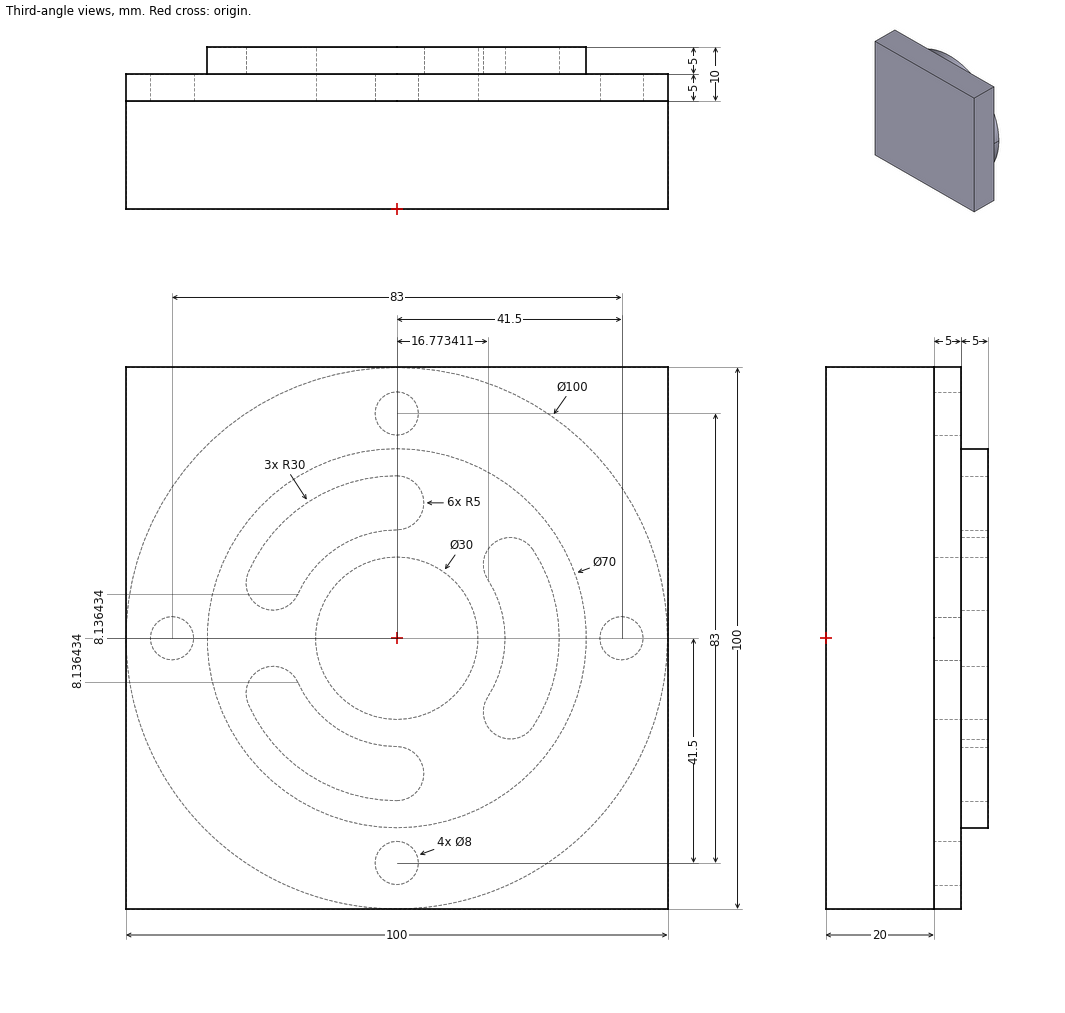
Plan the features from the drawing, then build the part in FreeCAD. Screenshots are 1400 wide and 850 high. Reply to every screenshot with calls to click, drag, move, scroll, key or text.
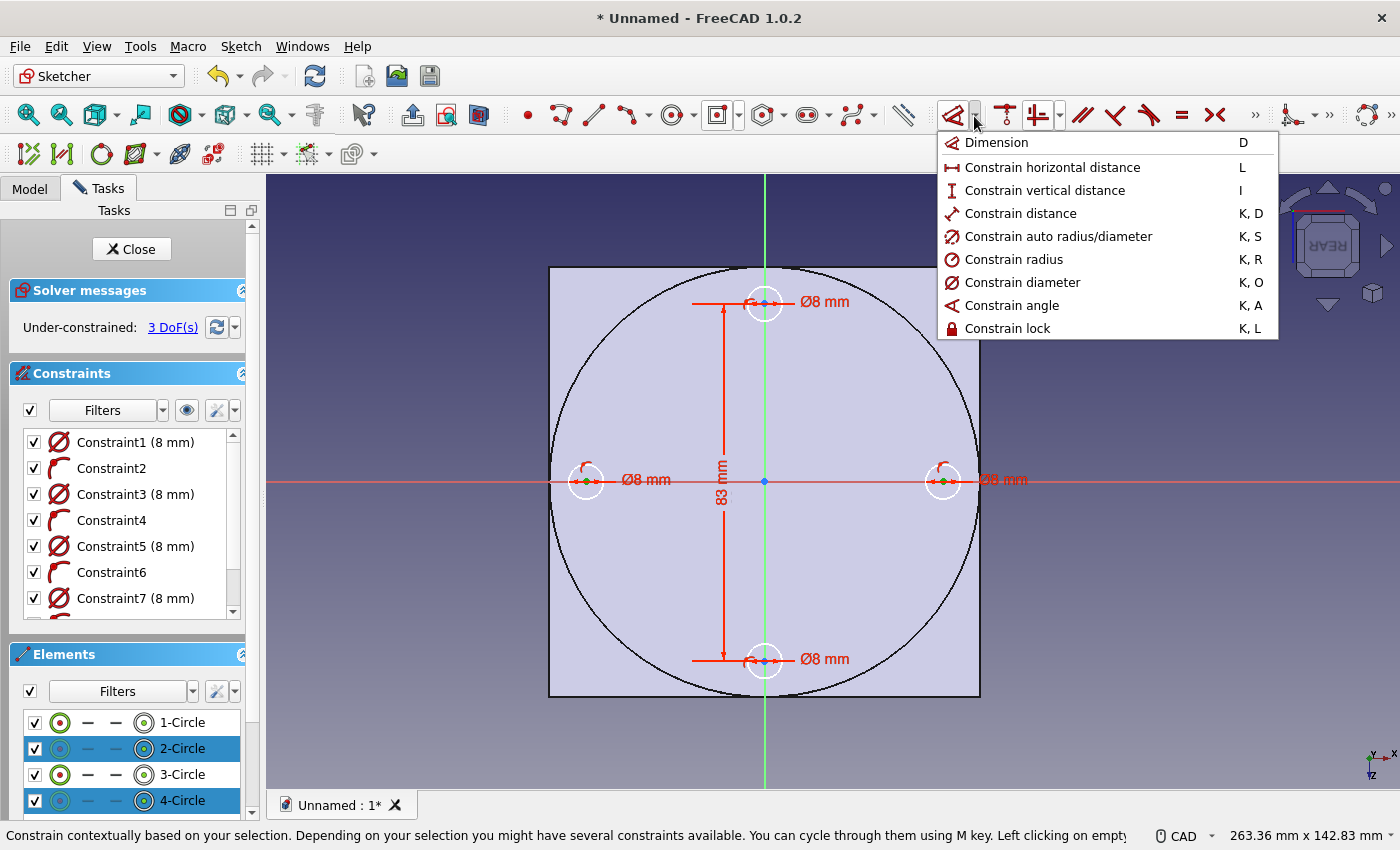
click(1108, 168)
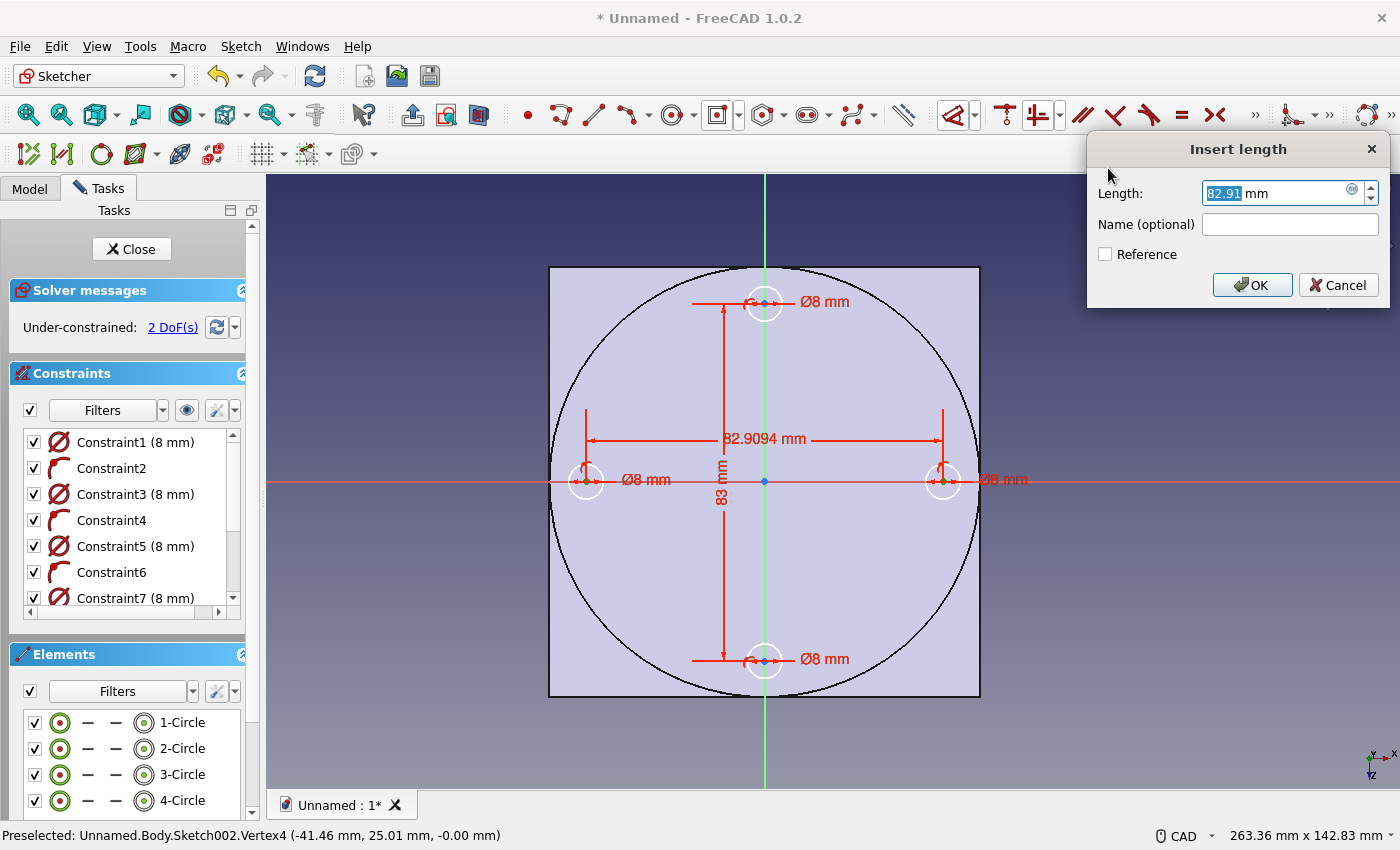
text(83)
key(Return)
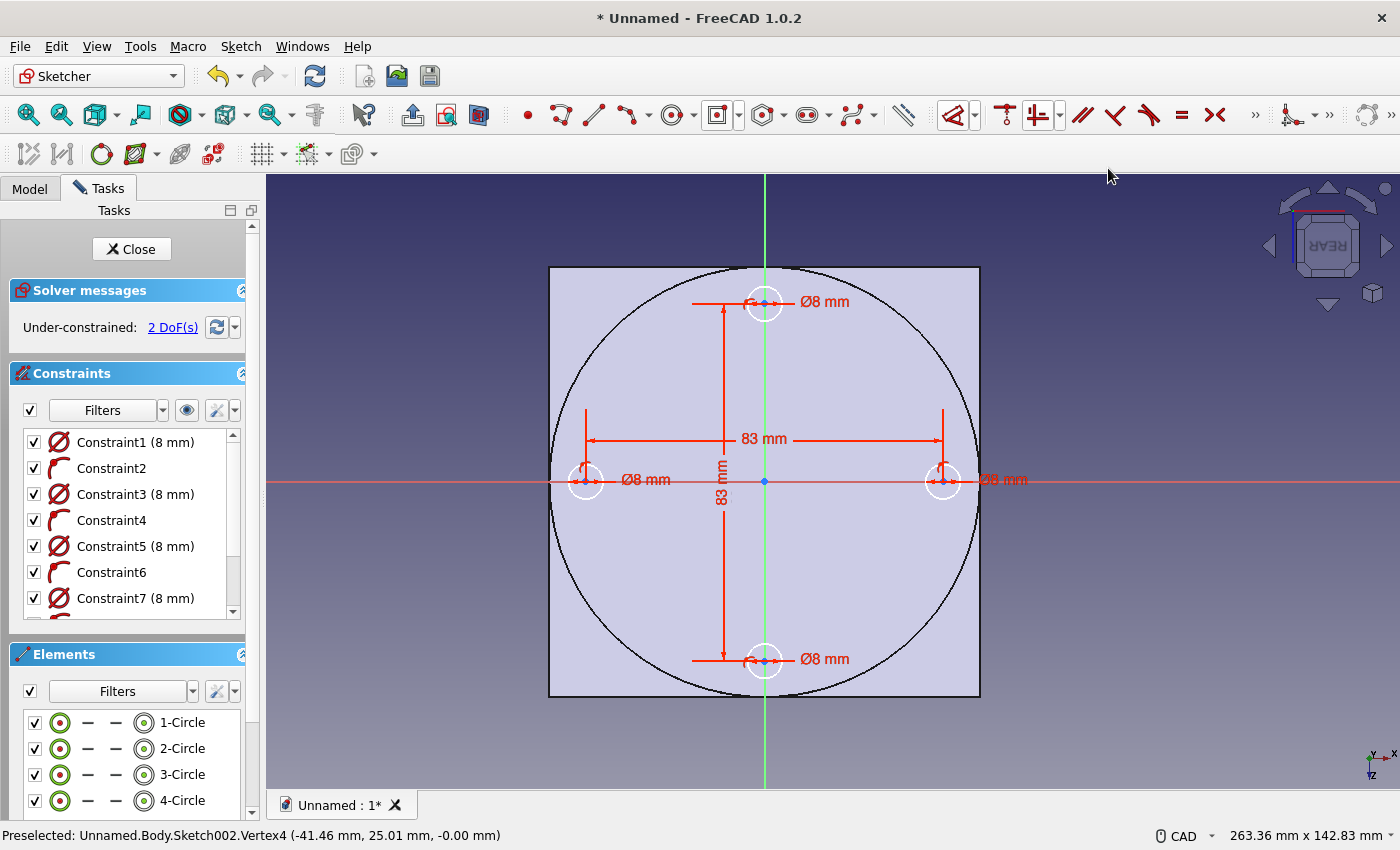
click(765, 304)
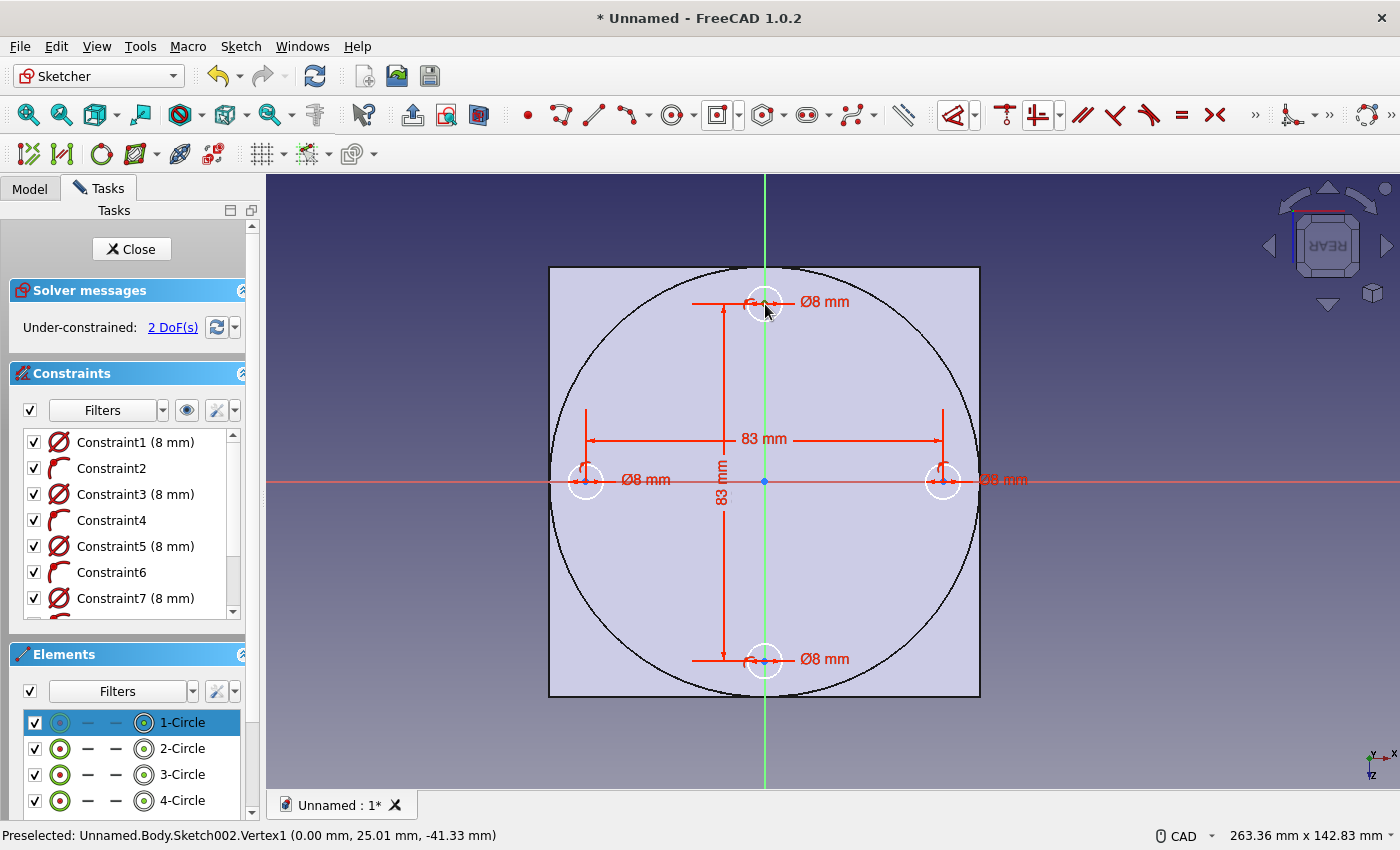
click(974, 116)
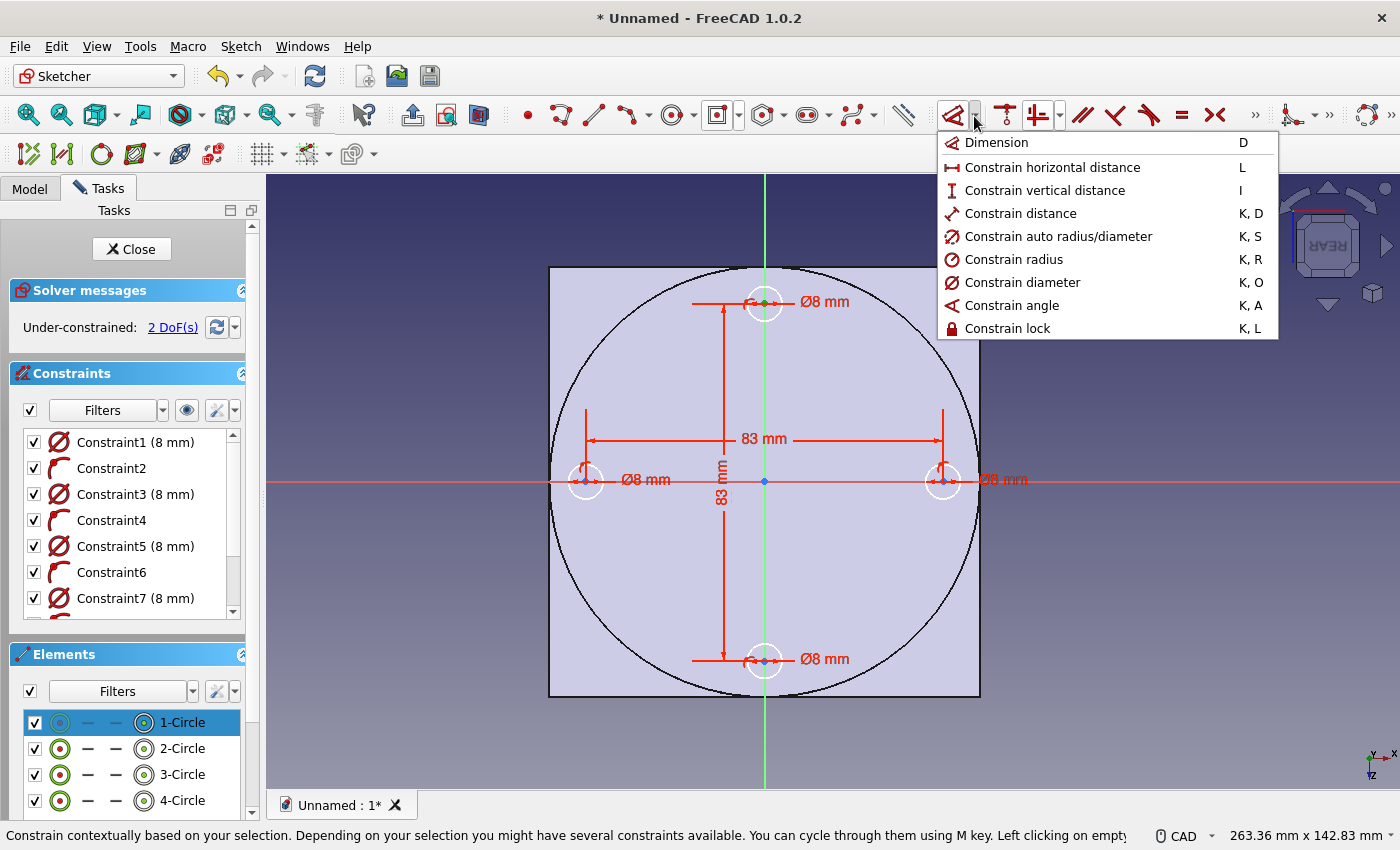
click(1108, 190)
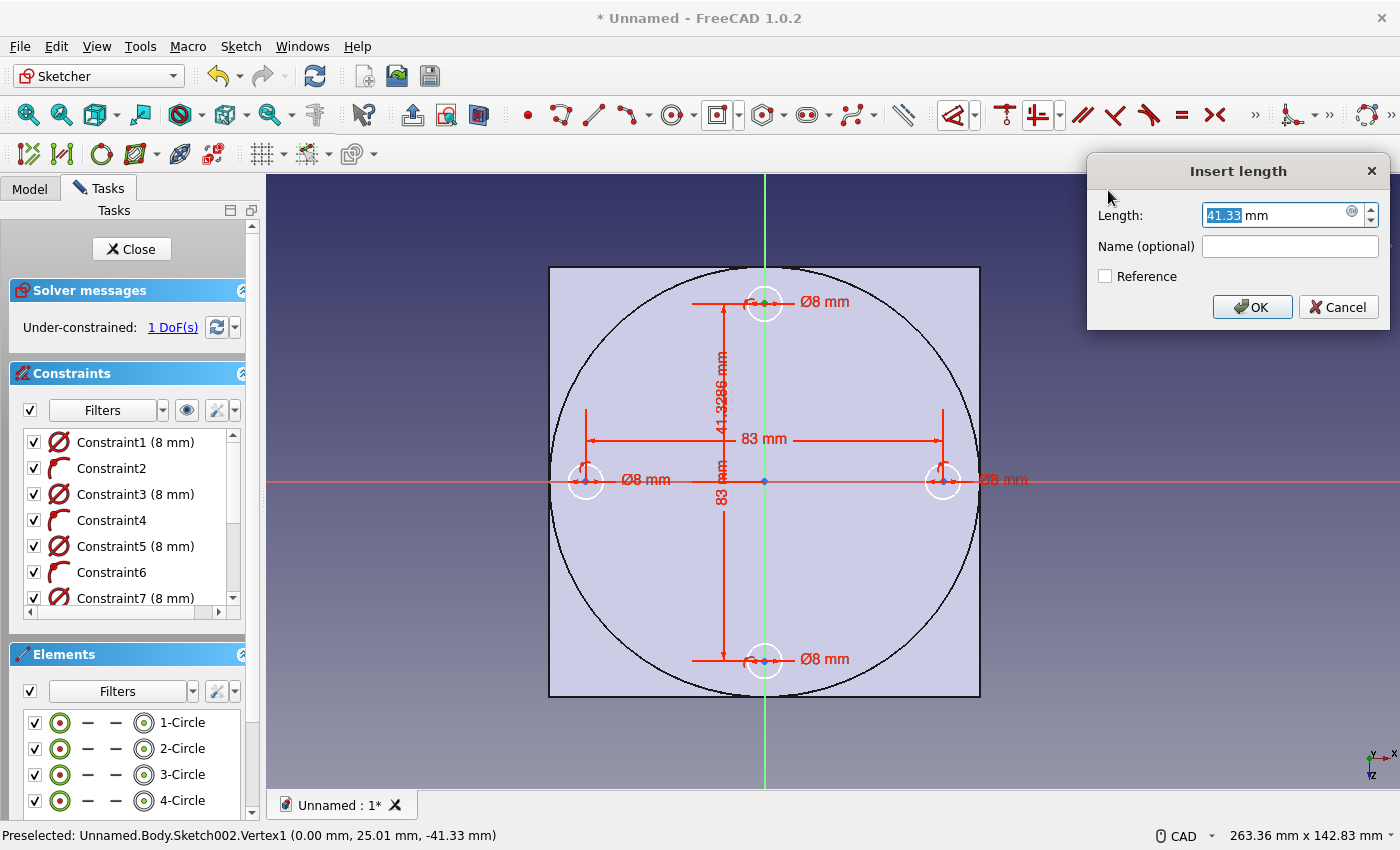
text(41.5)
key(Return)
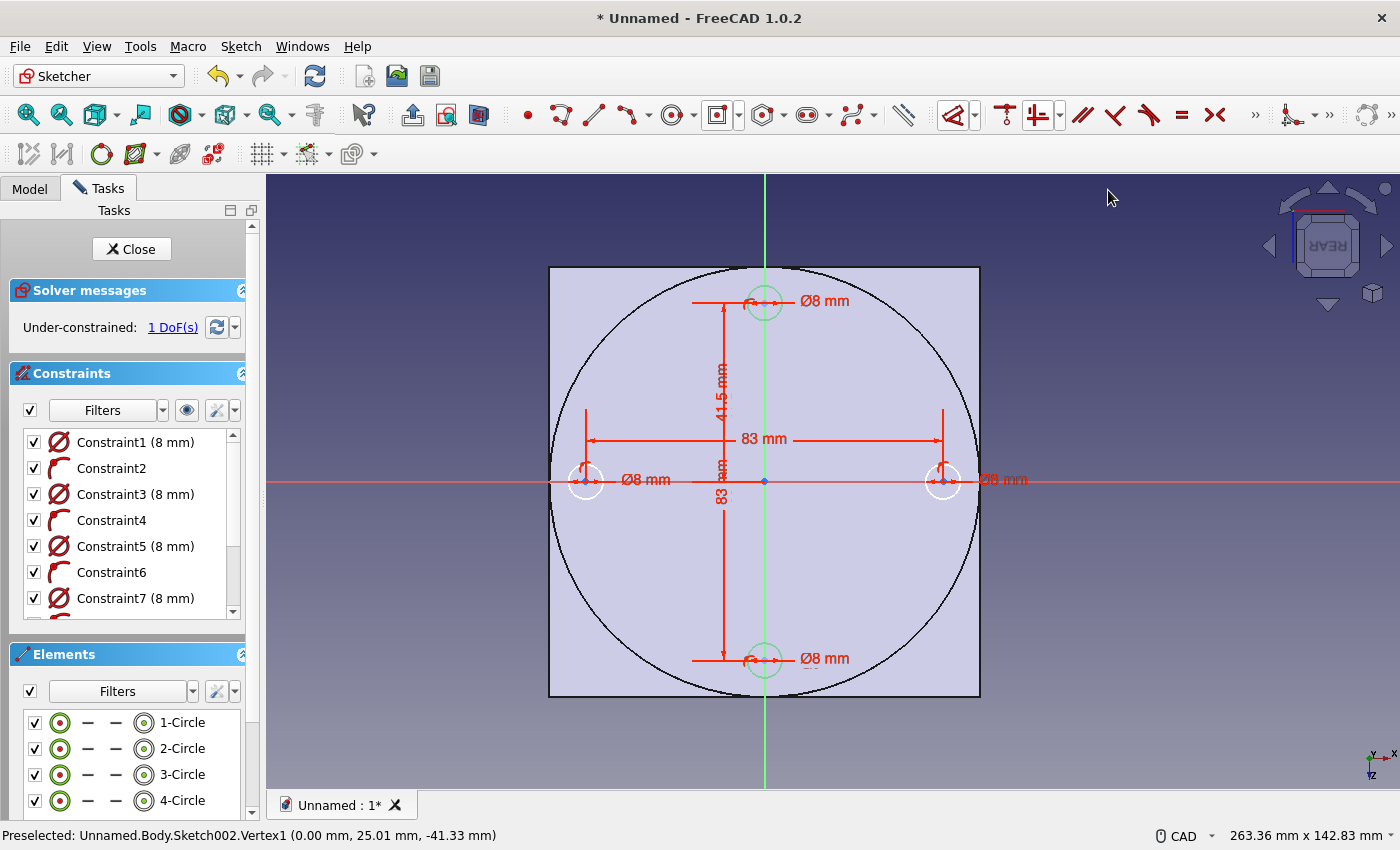
click(943, 482)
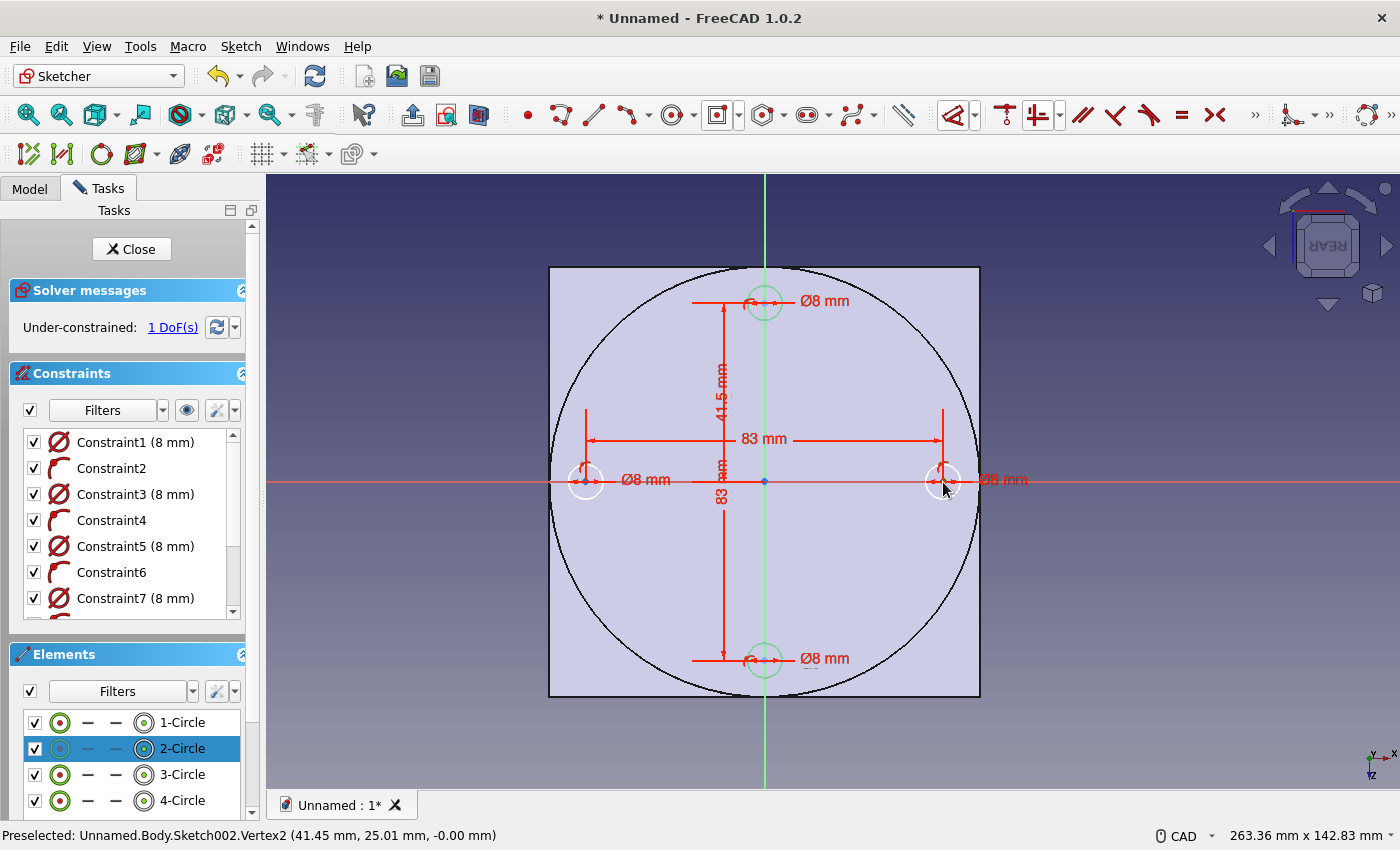
click(974, 116)